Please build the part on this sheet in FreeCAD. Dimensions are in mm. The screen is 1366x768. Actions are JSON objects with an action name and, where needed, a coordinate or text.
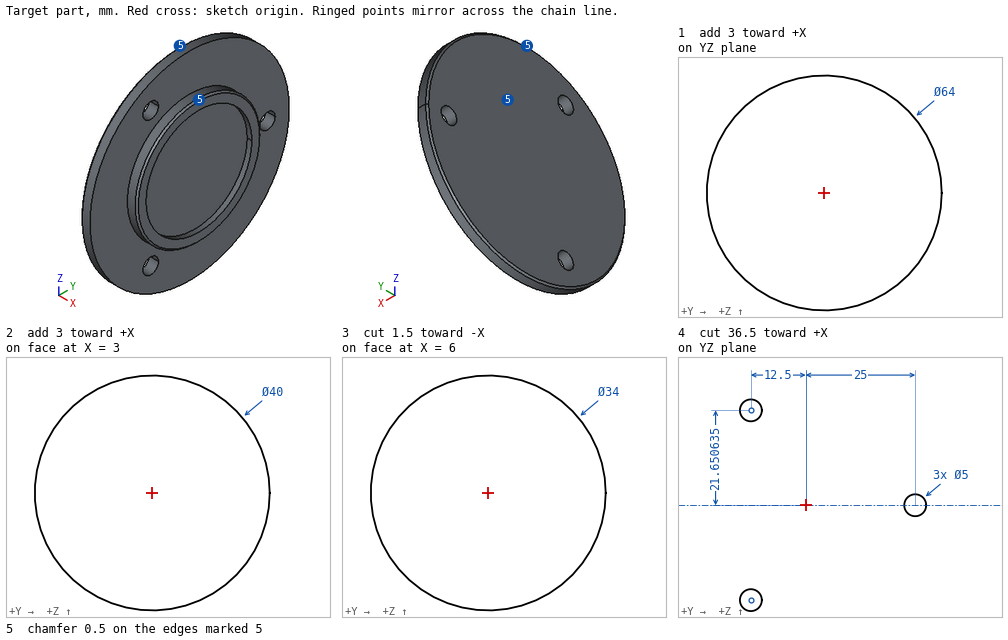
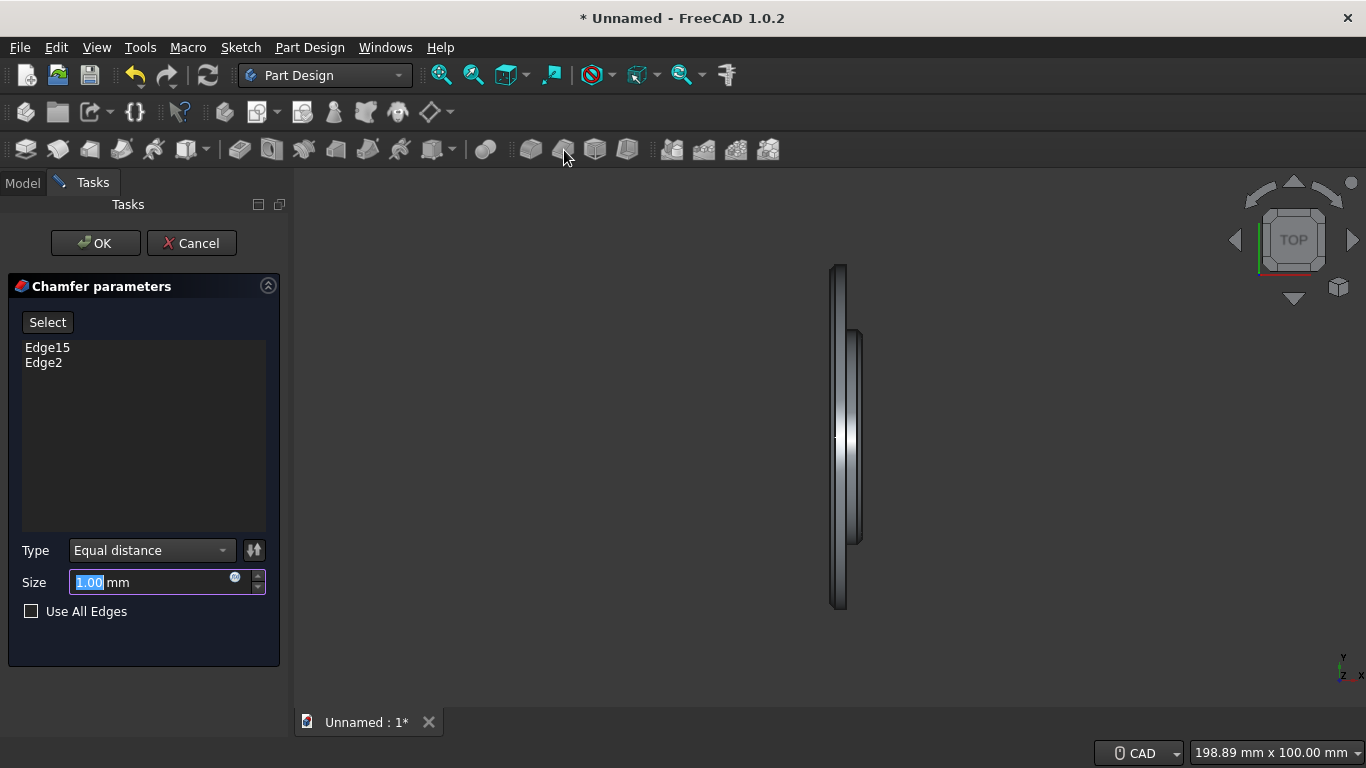
{"action": "type", "text": "0.5"}
{"action": "key", "text": "Tab"}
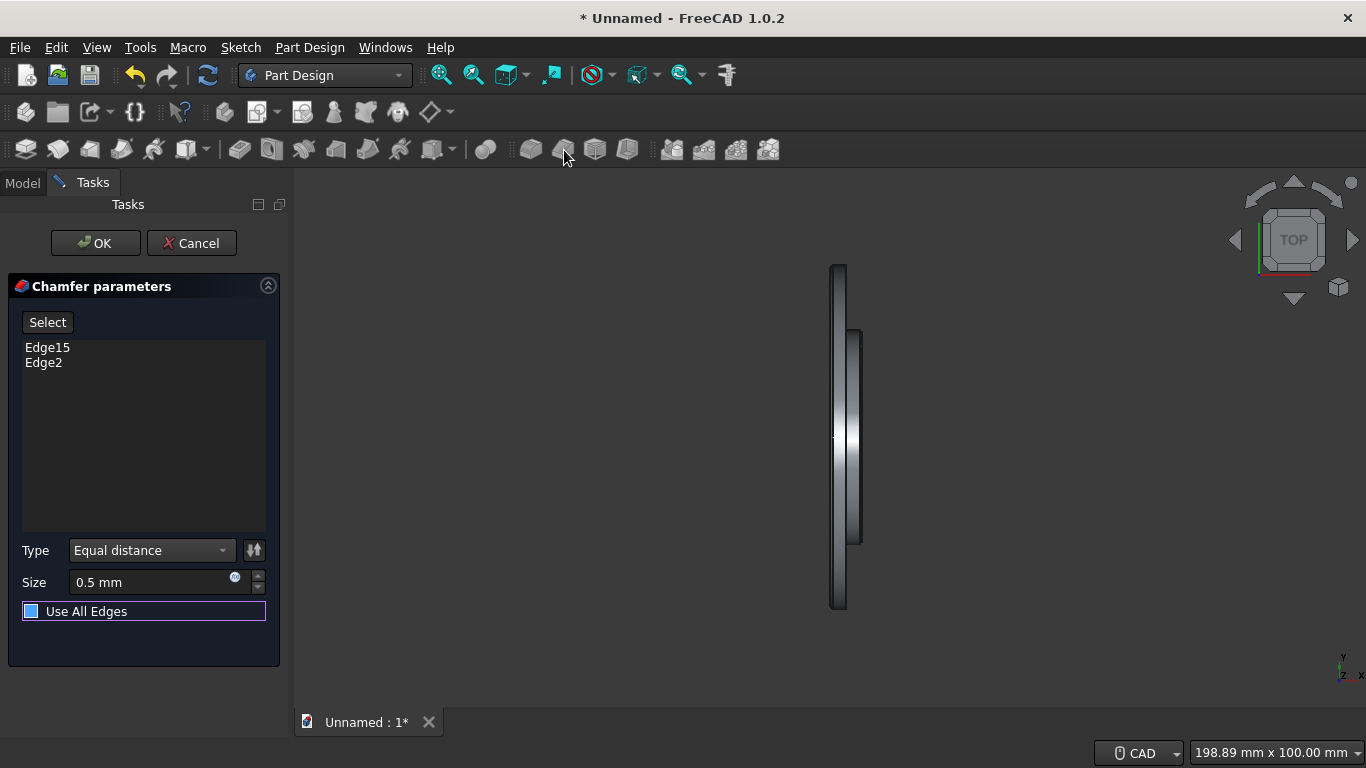
{"action": "left_click", "coordinate": [96, 243]}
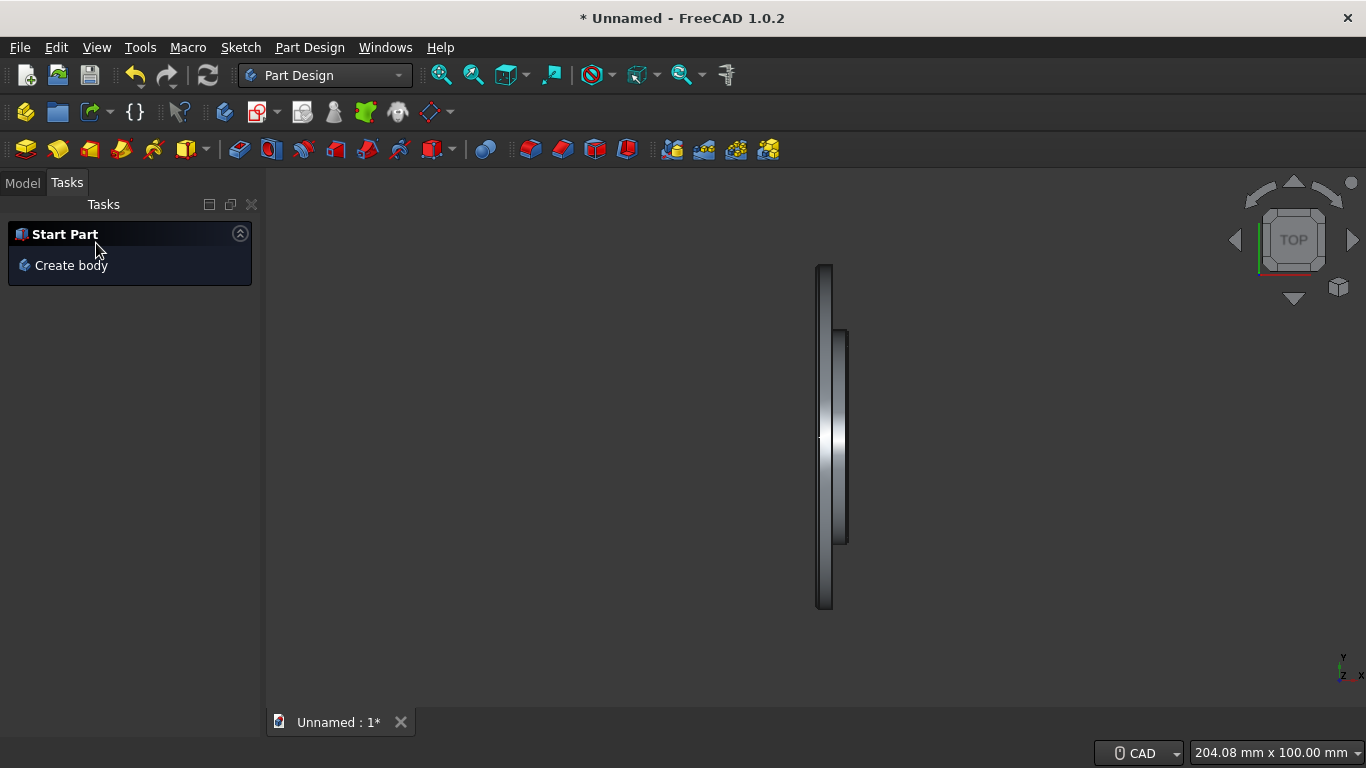
{"action": "key", "text": "0"}